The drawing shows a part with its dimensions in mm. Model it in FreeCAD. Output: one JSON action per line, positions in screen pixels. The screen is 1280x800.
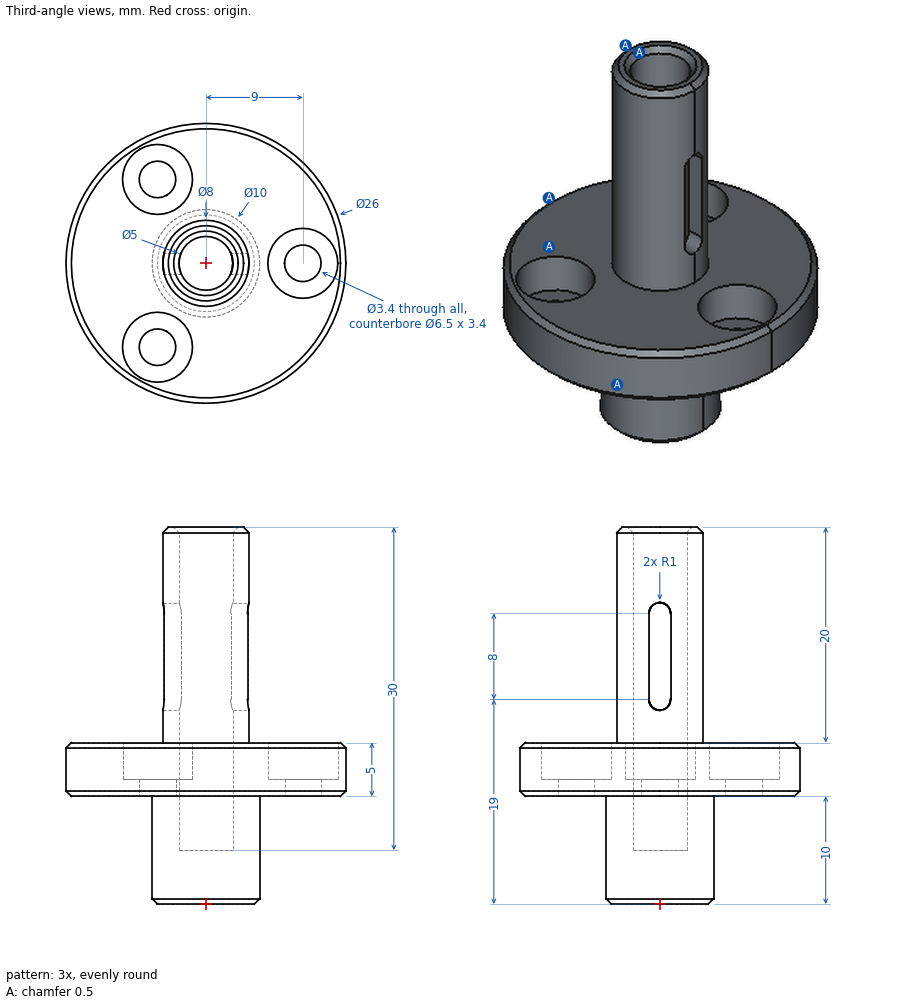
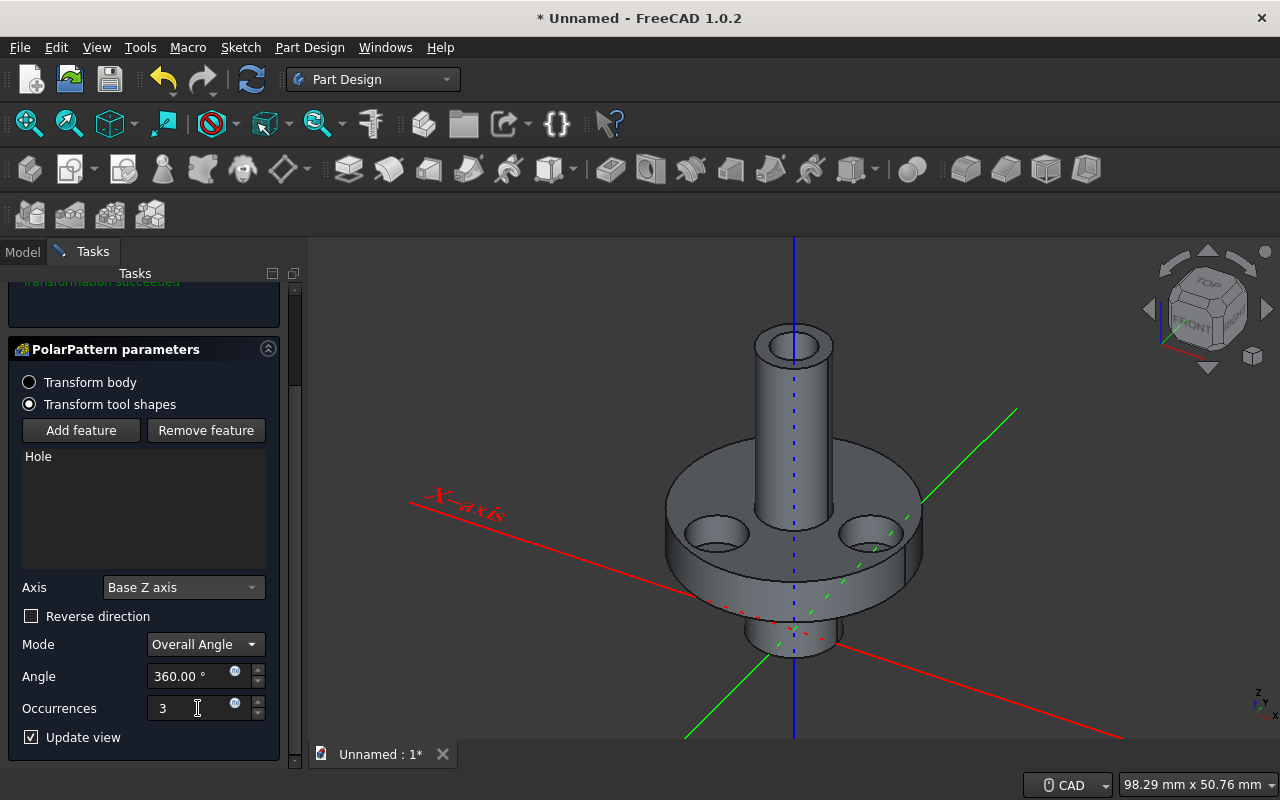
{"action": "scroll", "coordinate": [295, 526], "scroll_direction": "up", "scroll_amount": 3}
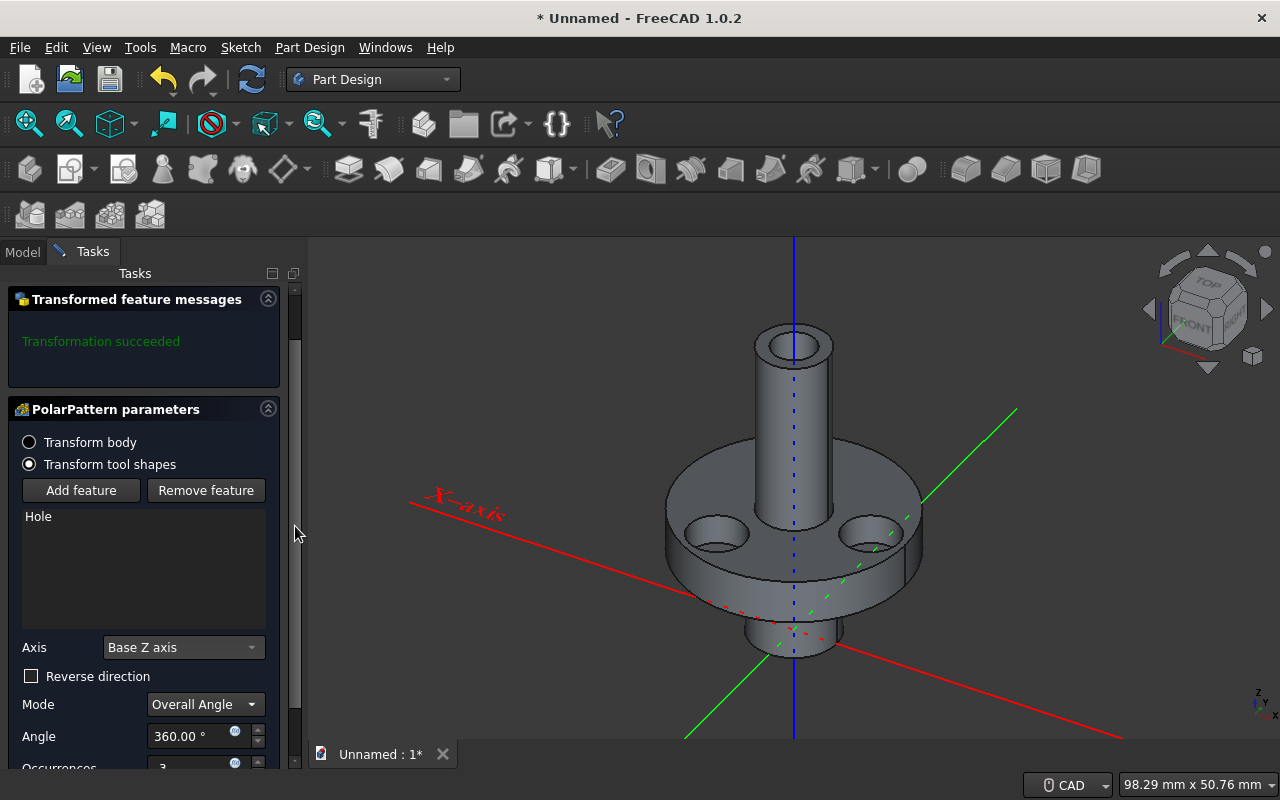
{"action": "left_click", "coordinate": [96, 312]}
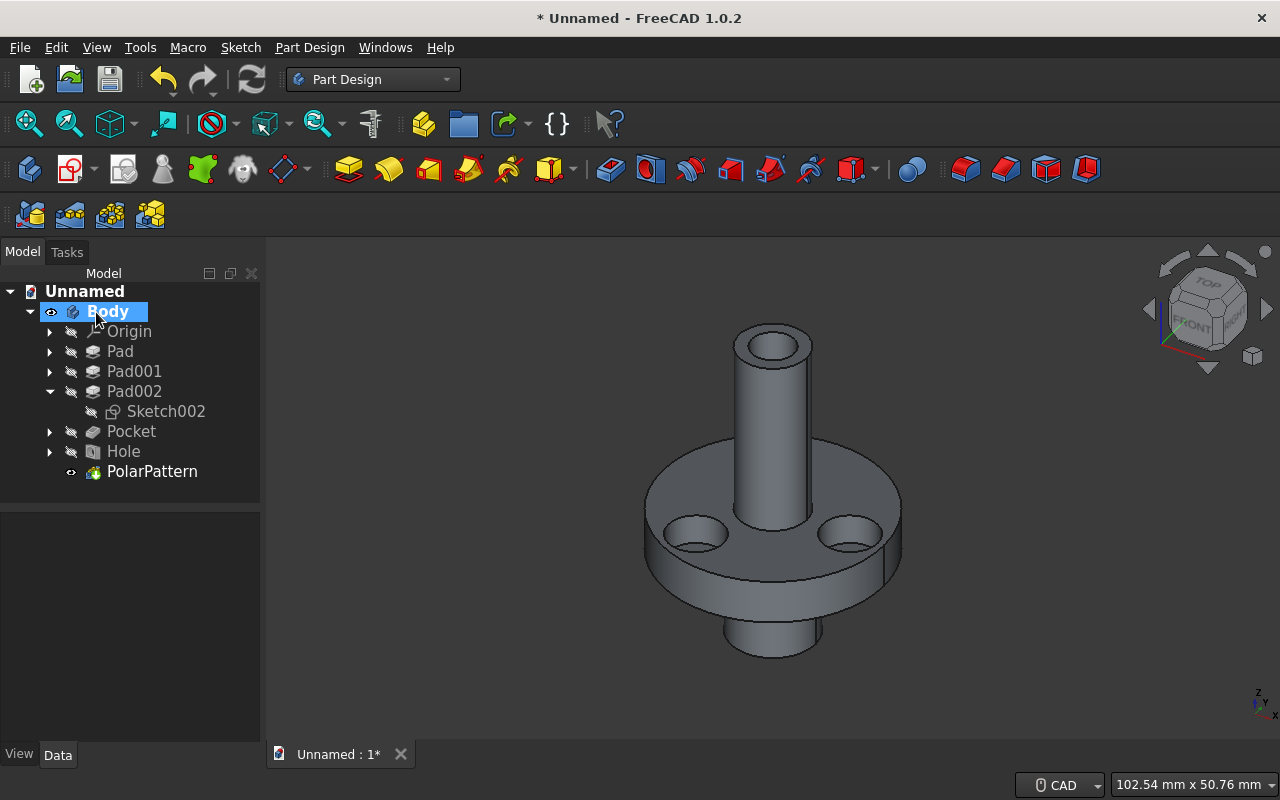
{"action": "left_click", "coordinate": [50, 332]}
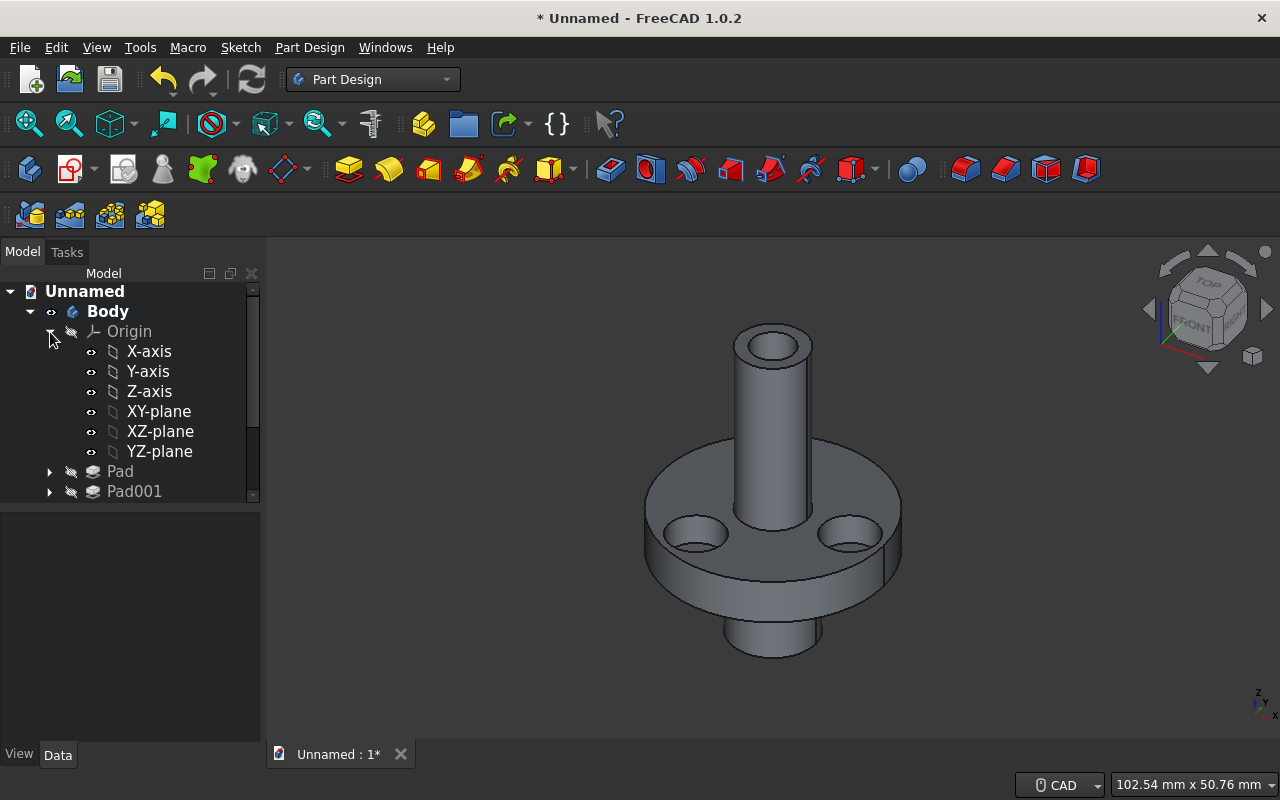
{"action": "left_click", "coordinate": [136, 452]}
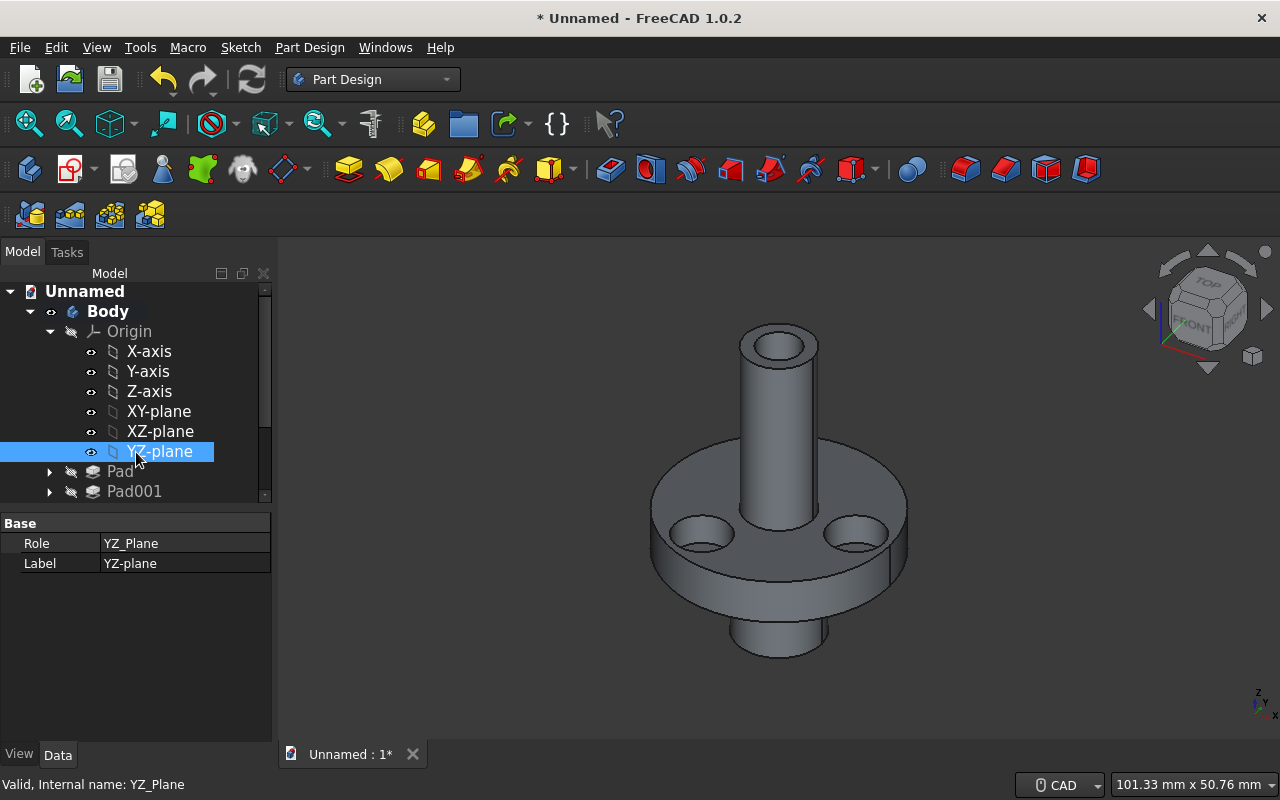
{"action": "left_click", "coordinate": [284, 170]}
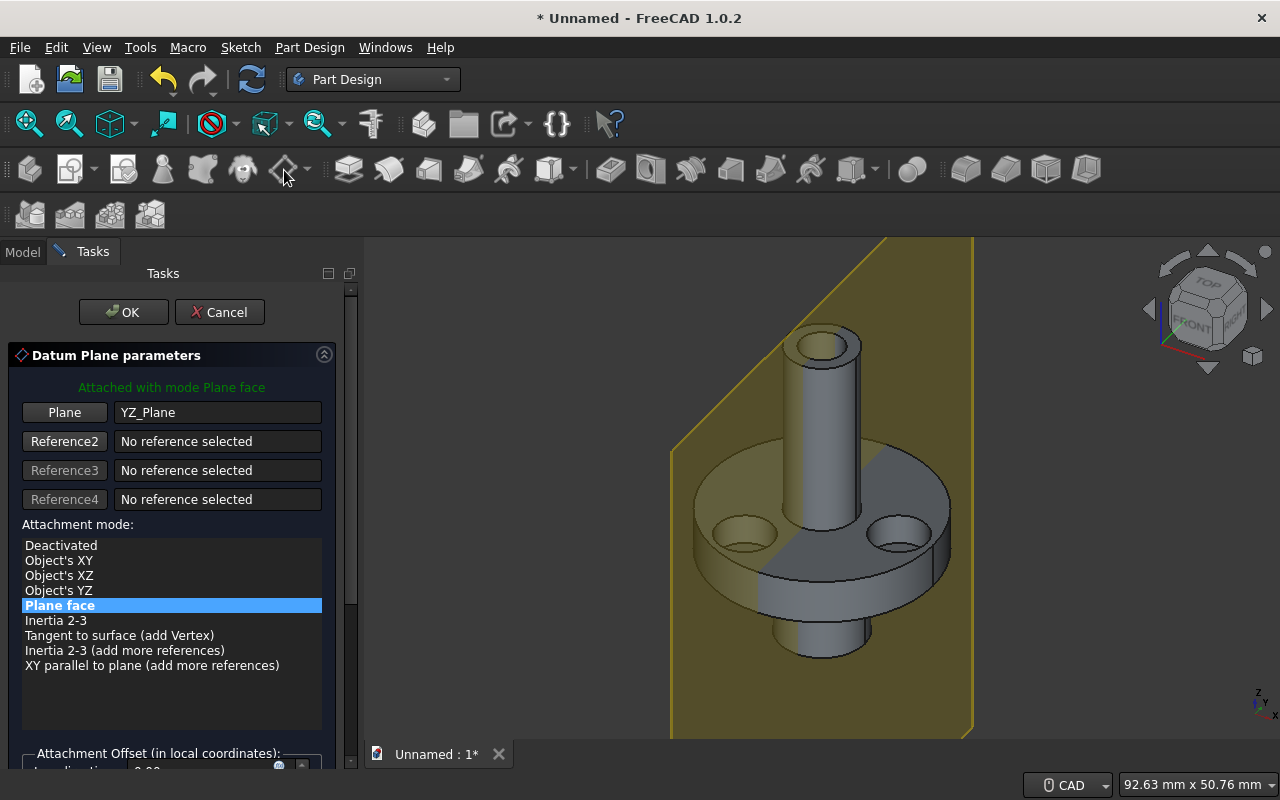
{"action": "scroll", "coordinate": [351, 526], "scroll_direction": "down", "scroll_amount": 3}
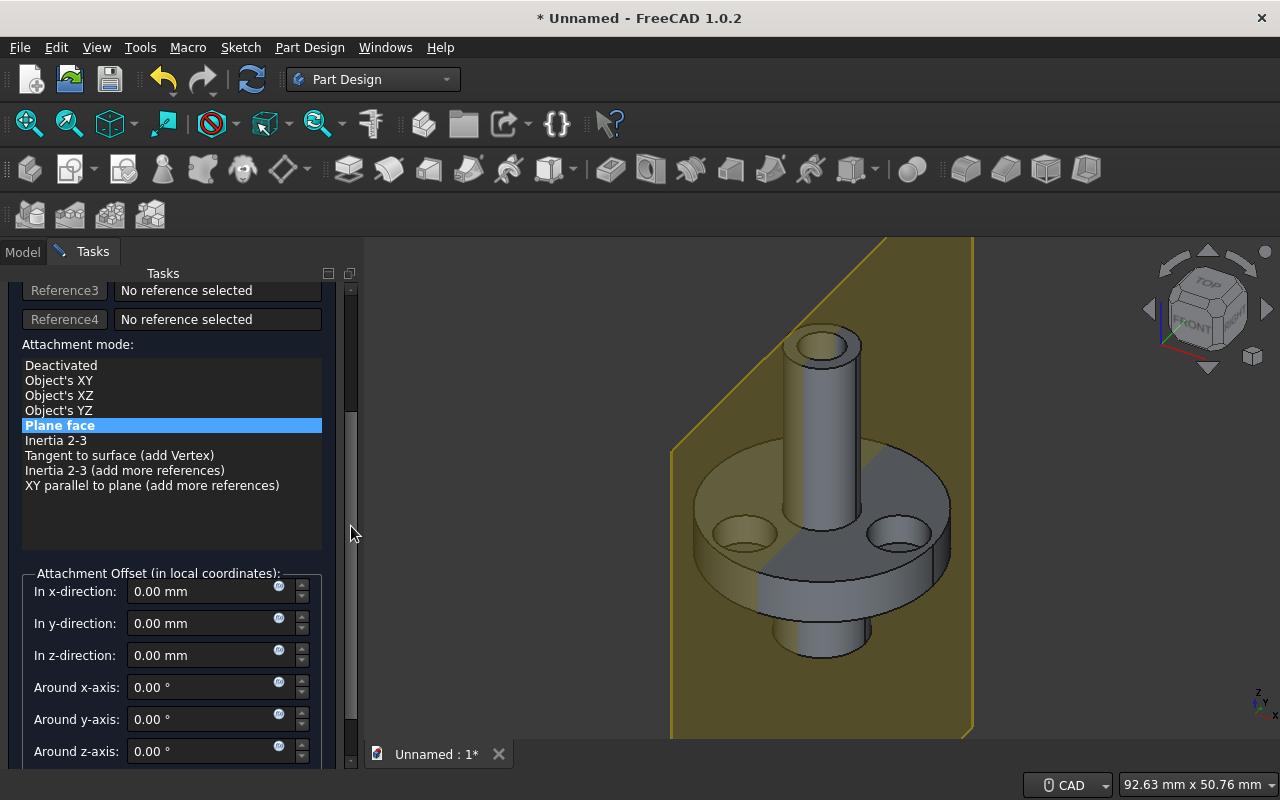
{"action": "triple_click", "coordinate": [210, 655]}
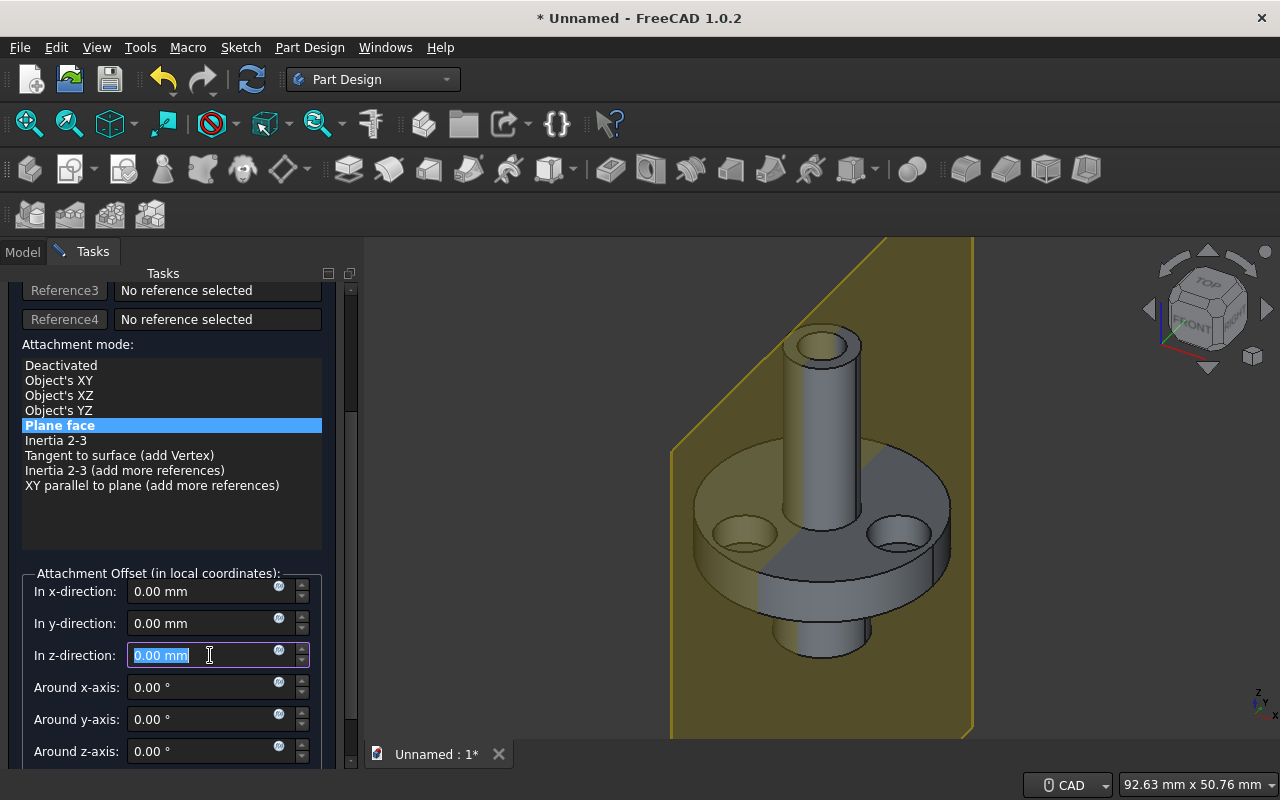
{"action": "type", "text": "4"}
{"action": "key", "text": "Tab"}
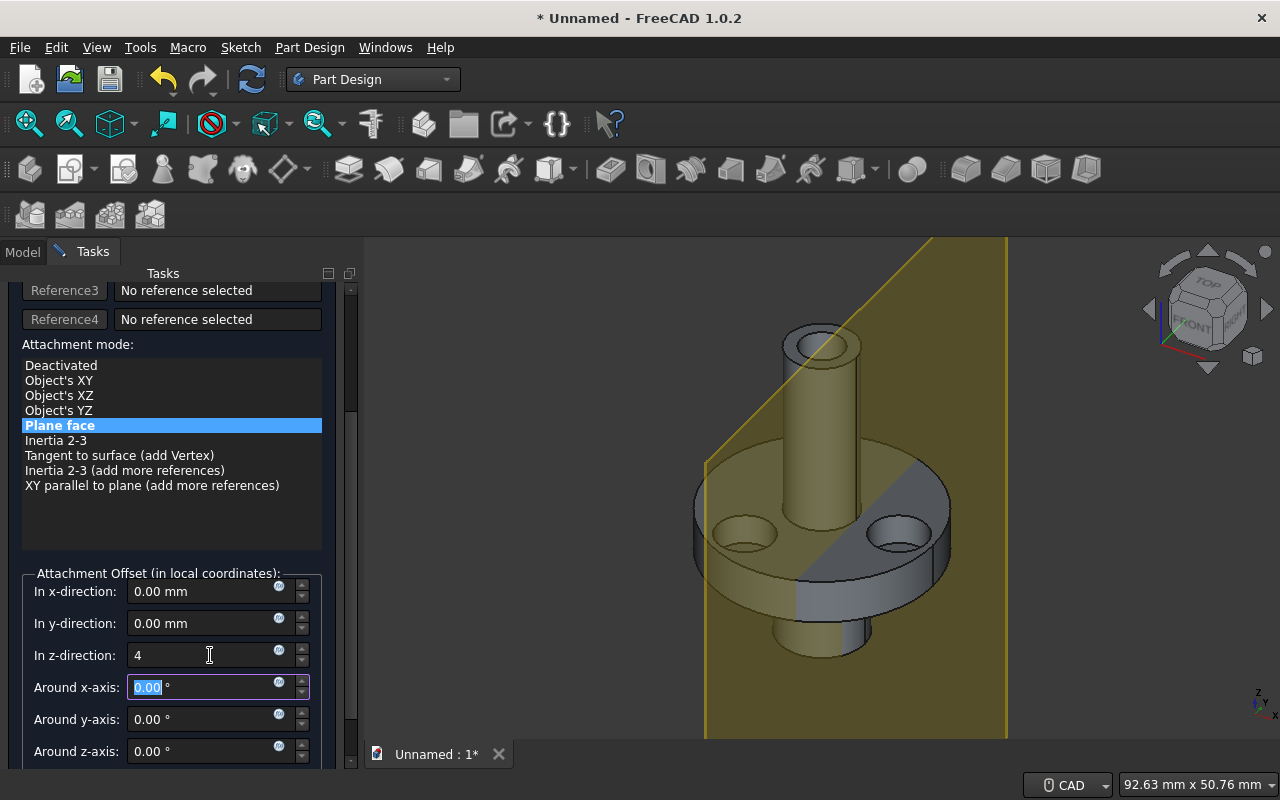
{"action": "scroll", "coordinate": [351, 526], "scroll_direction": "up", "scroll_amount": 4}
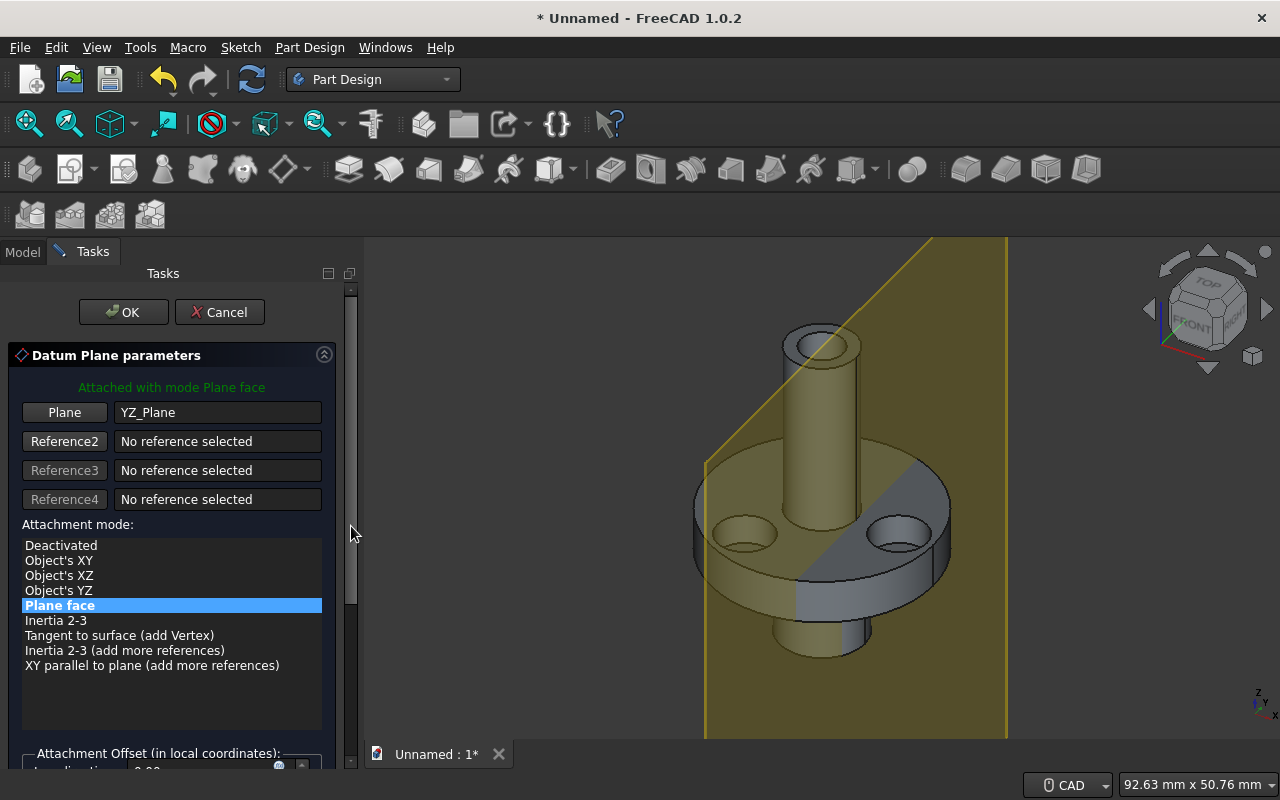
{"action": "left_click", "coordinate": [124, 312]}